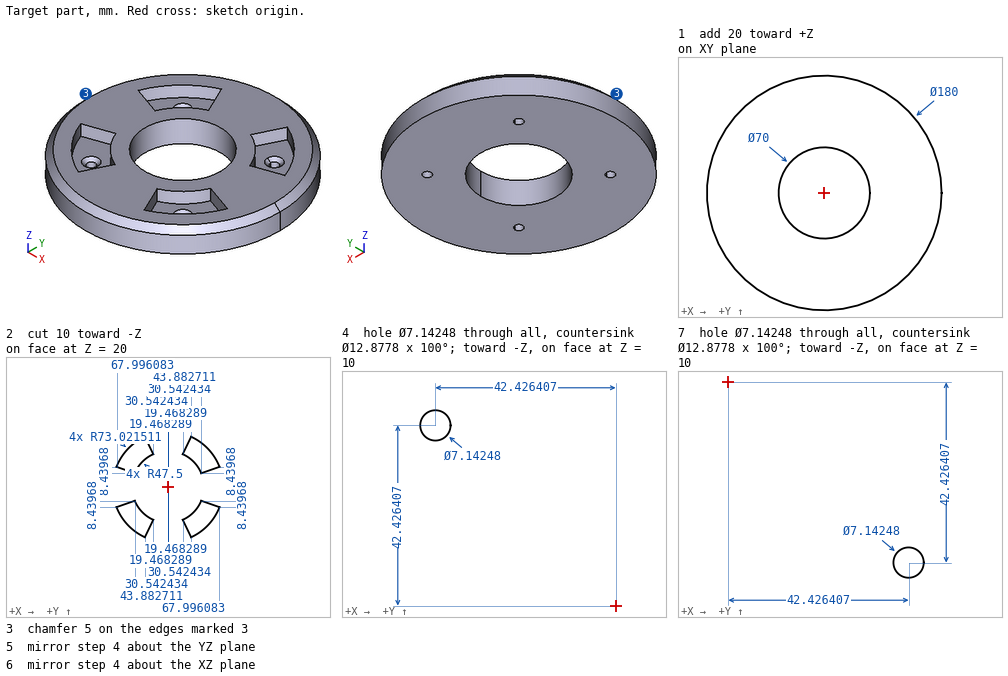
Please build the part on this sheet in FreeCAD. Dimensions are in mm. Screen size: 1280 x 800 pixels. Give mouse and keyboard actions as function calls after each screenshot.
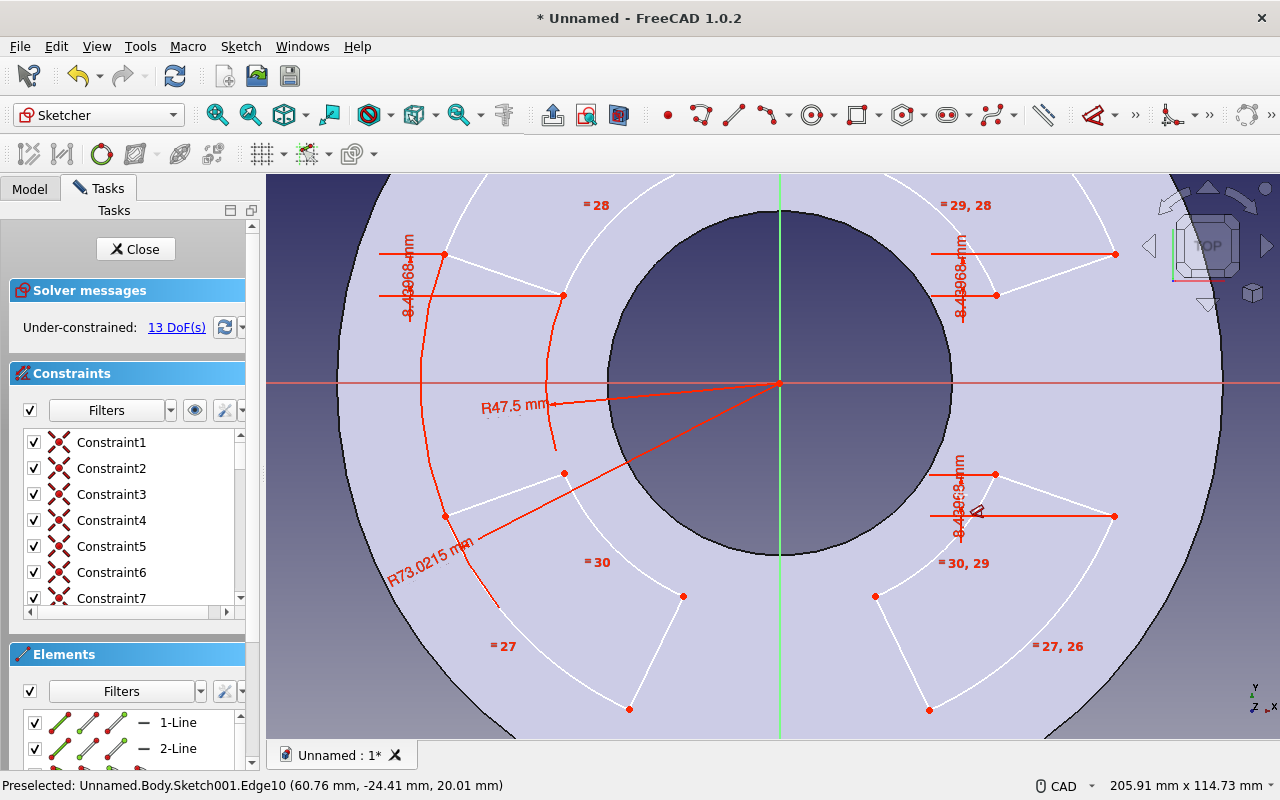
click(529, 487)
click(412, 495)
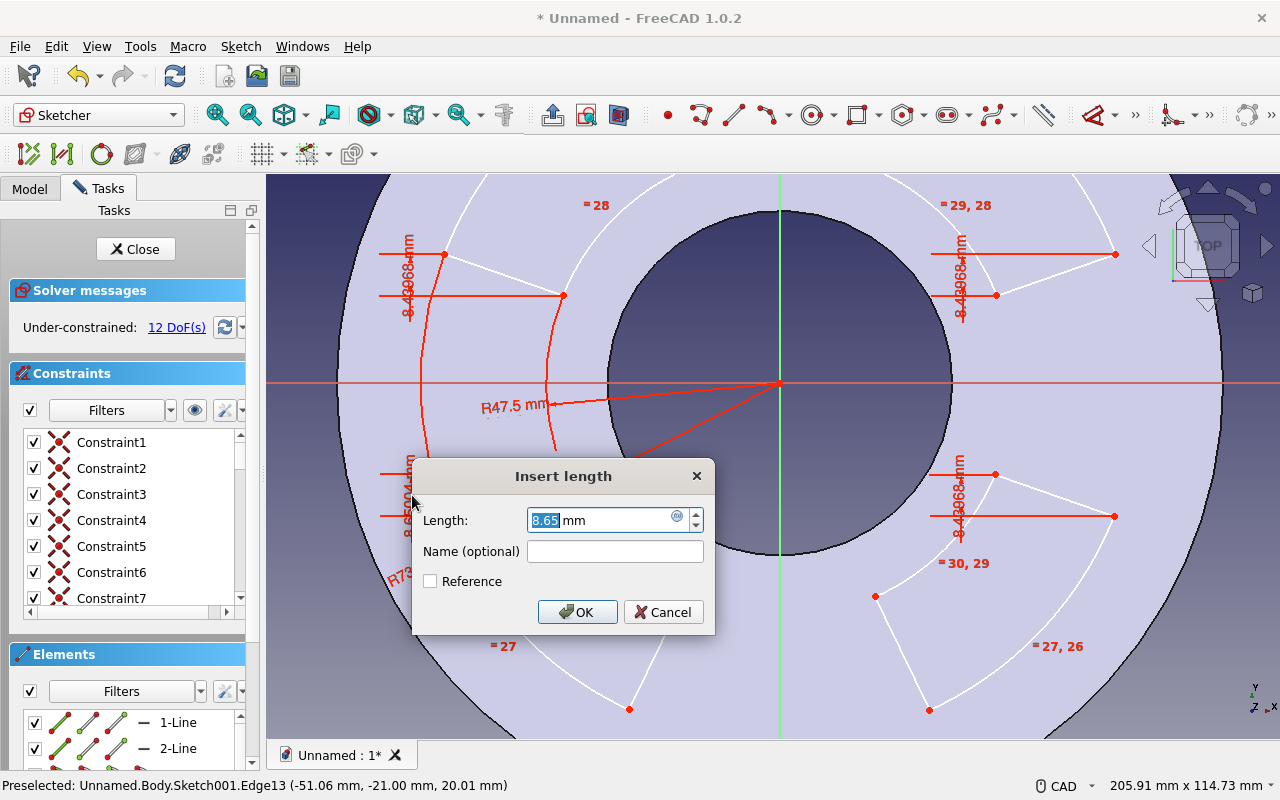
text(8.43968)
key(Return)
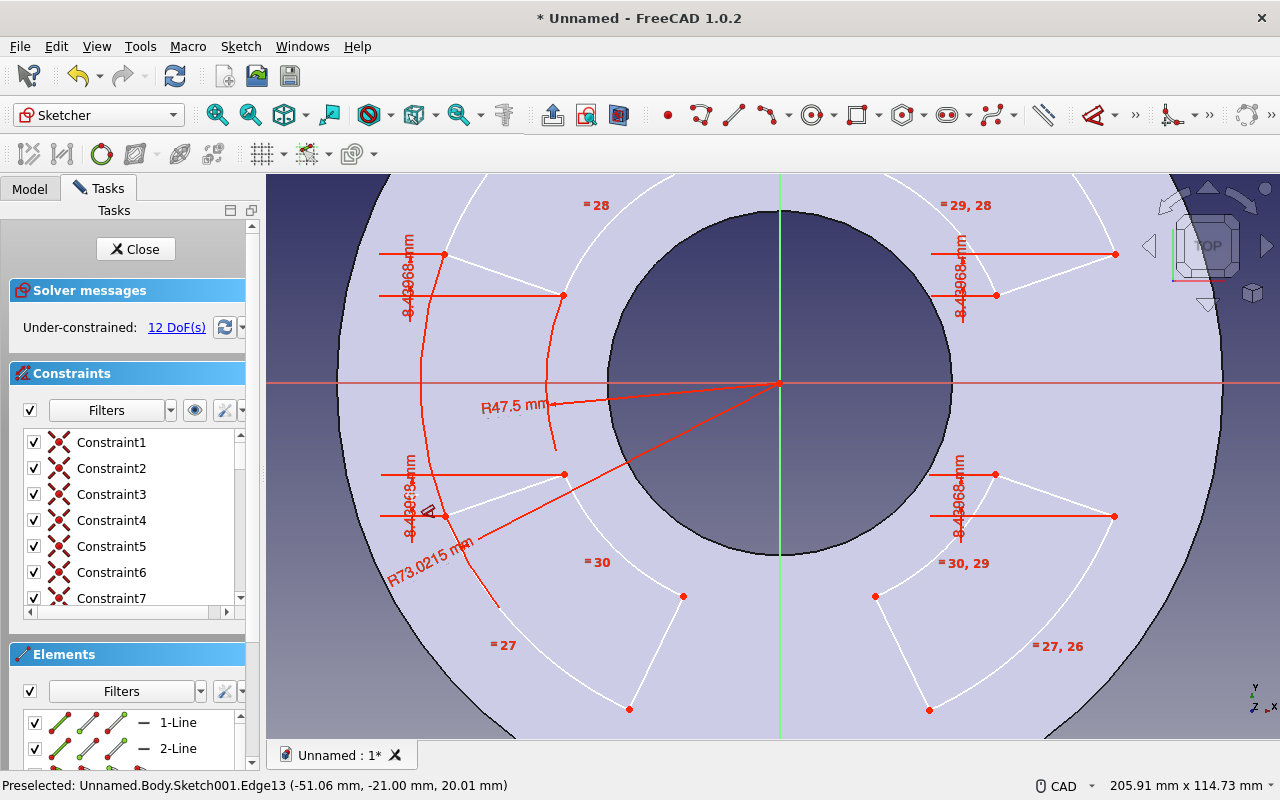
scroll(613, 546, down, 3)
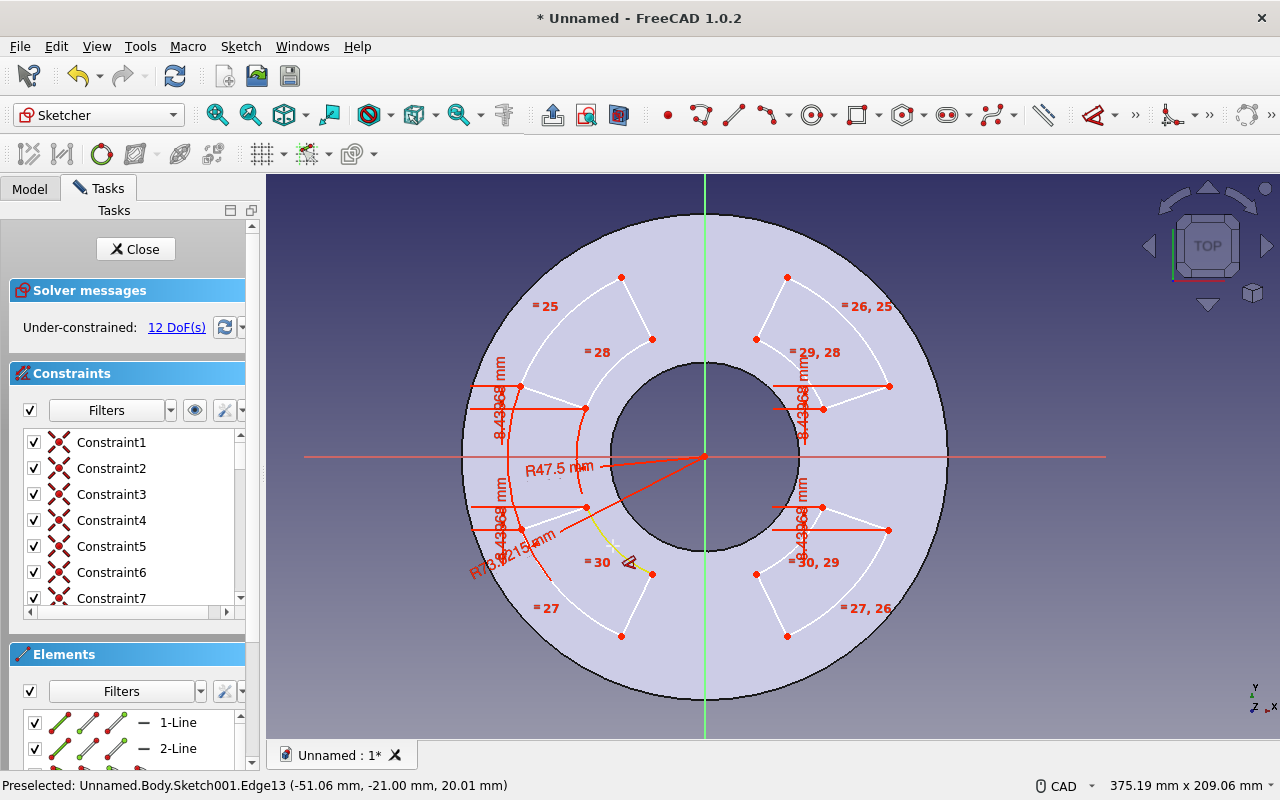
click(652, 340)
click(679, 306)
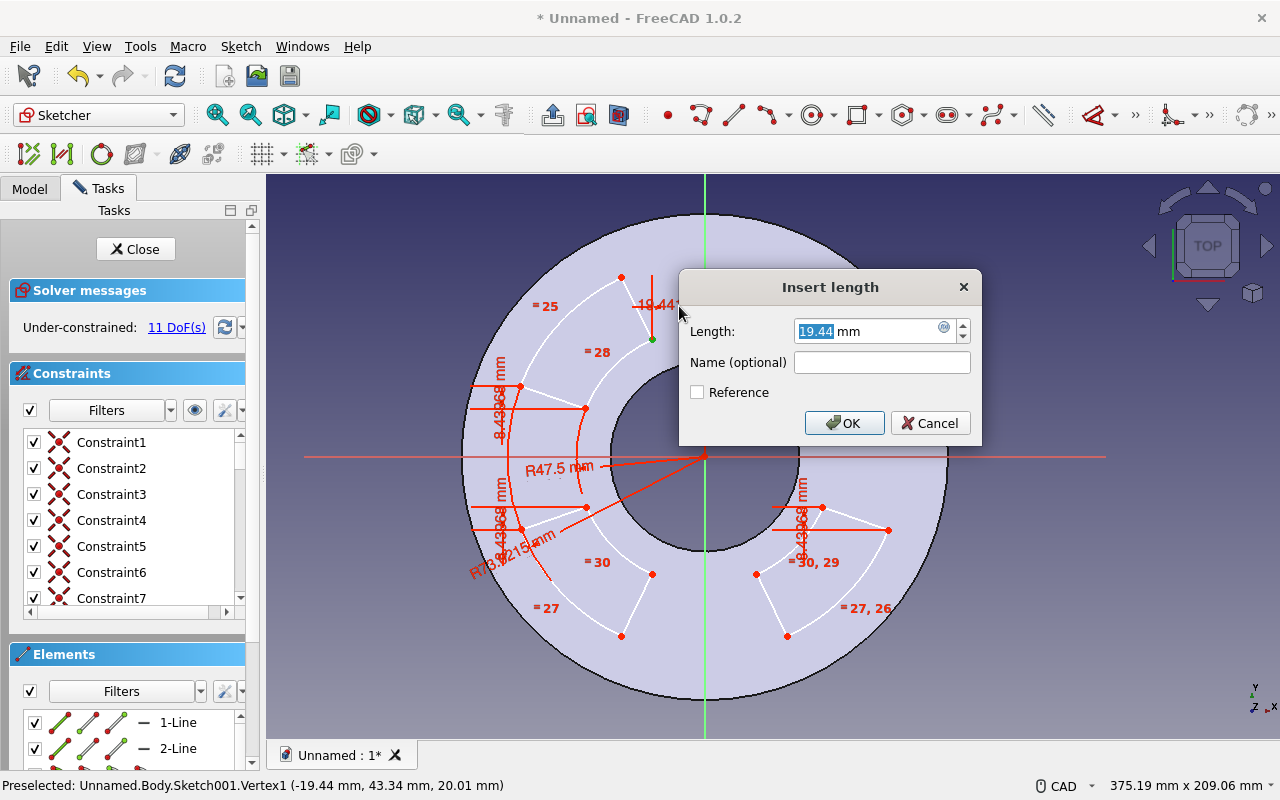
text(19.468289)
key(Return)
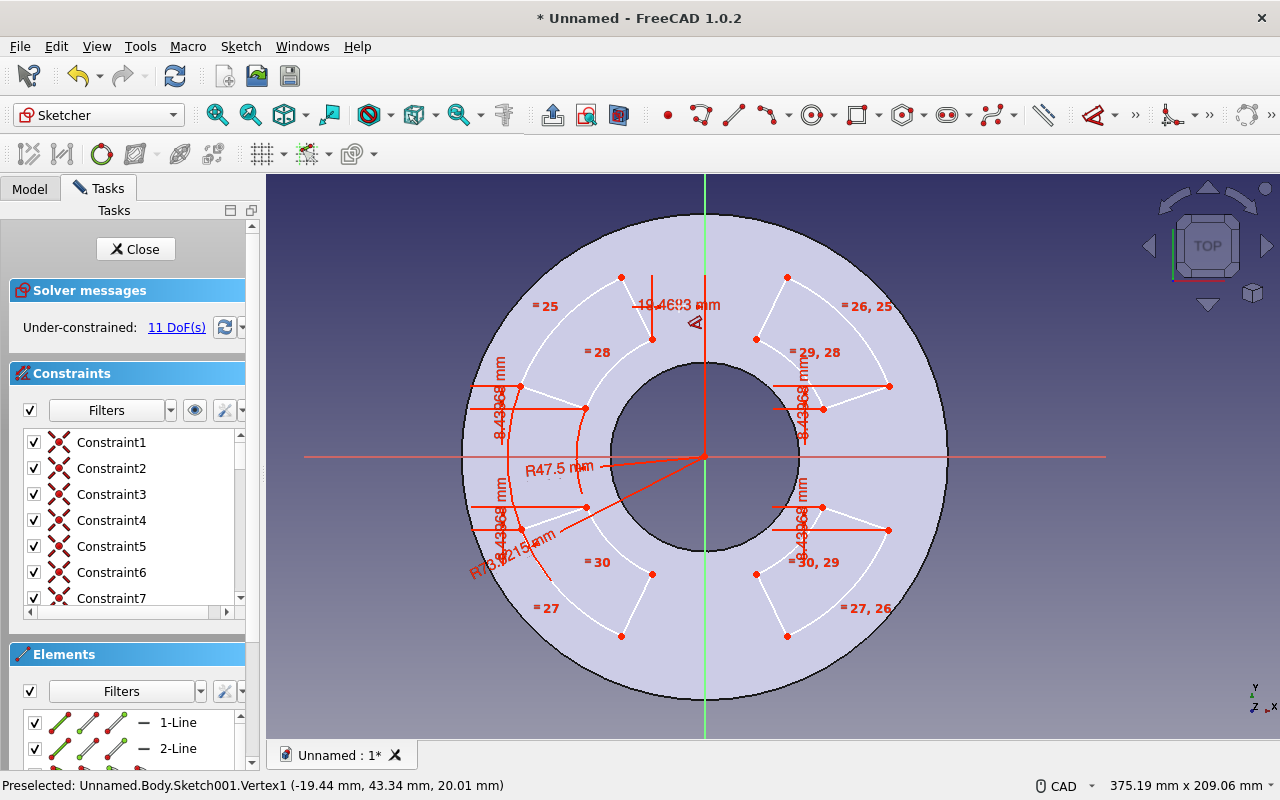
click(622, 278)
click(663, 244)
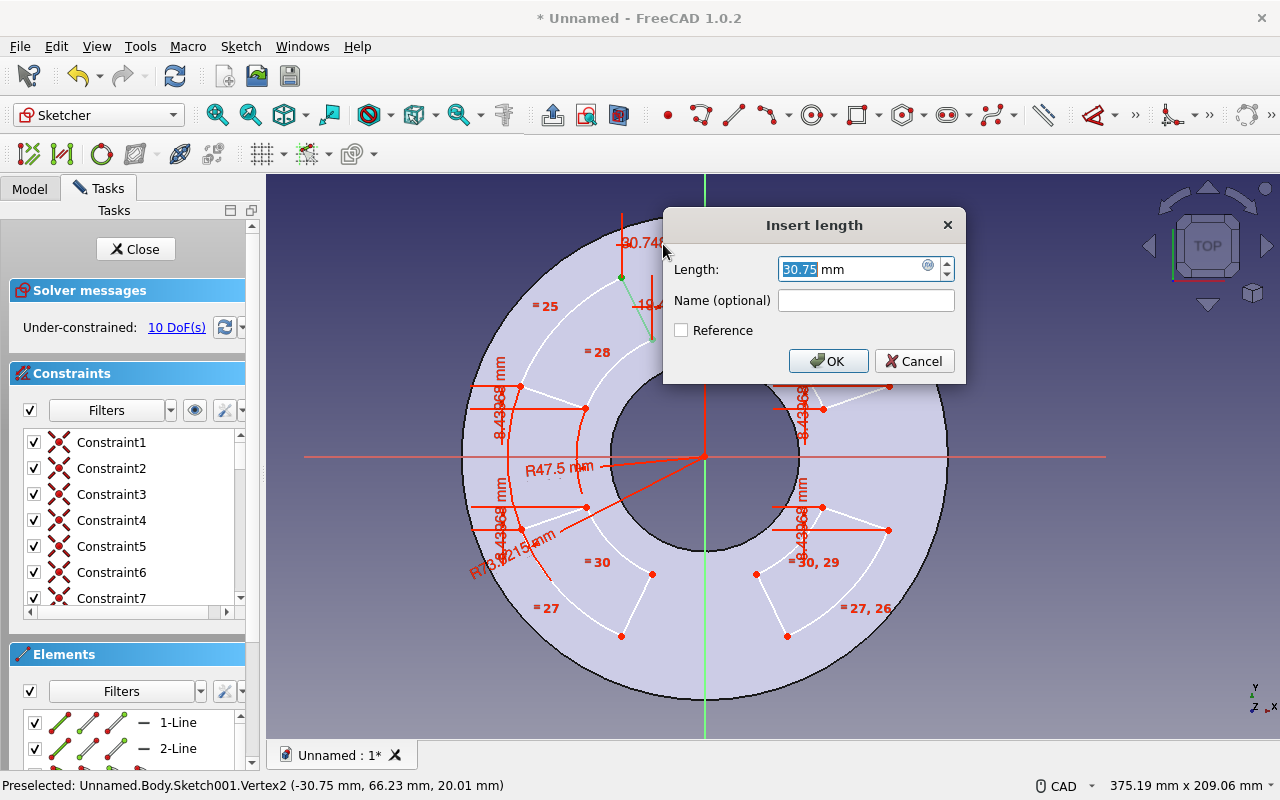
text(30.542434)
key(Return)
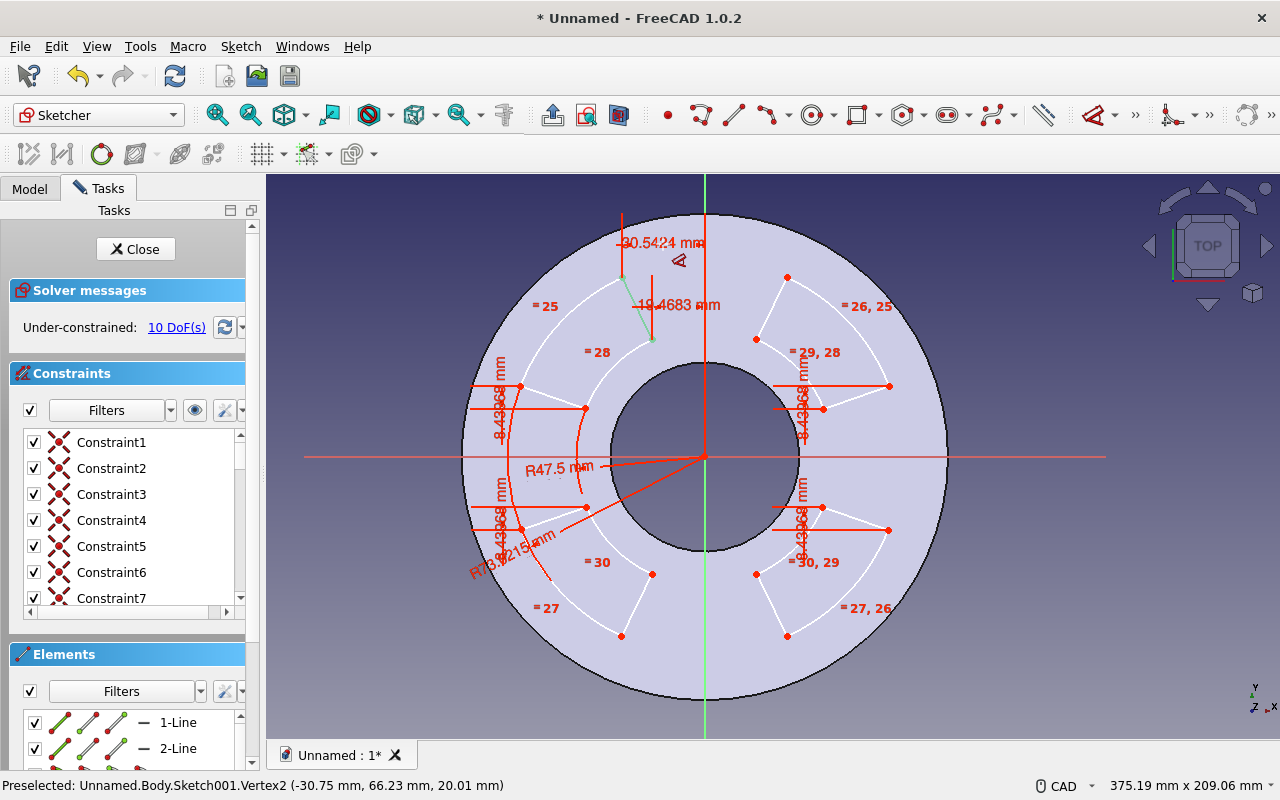
click(521, 386)
click(570, 352)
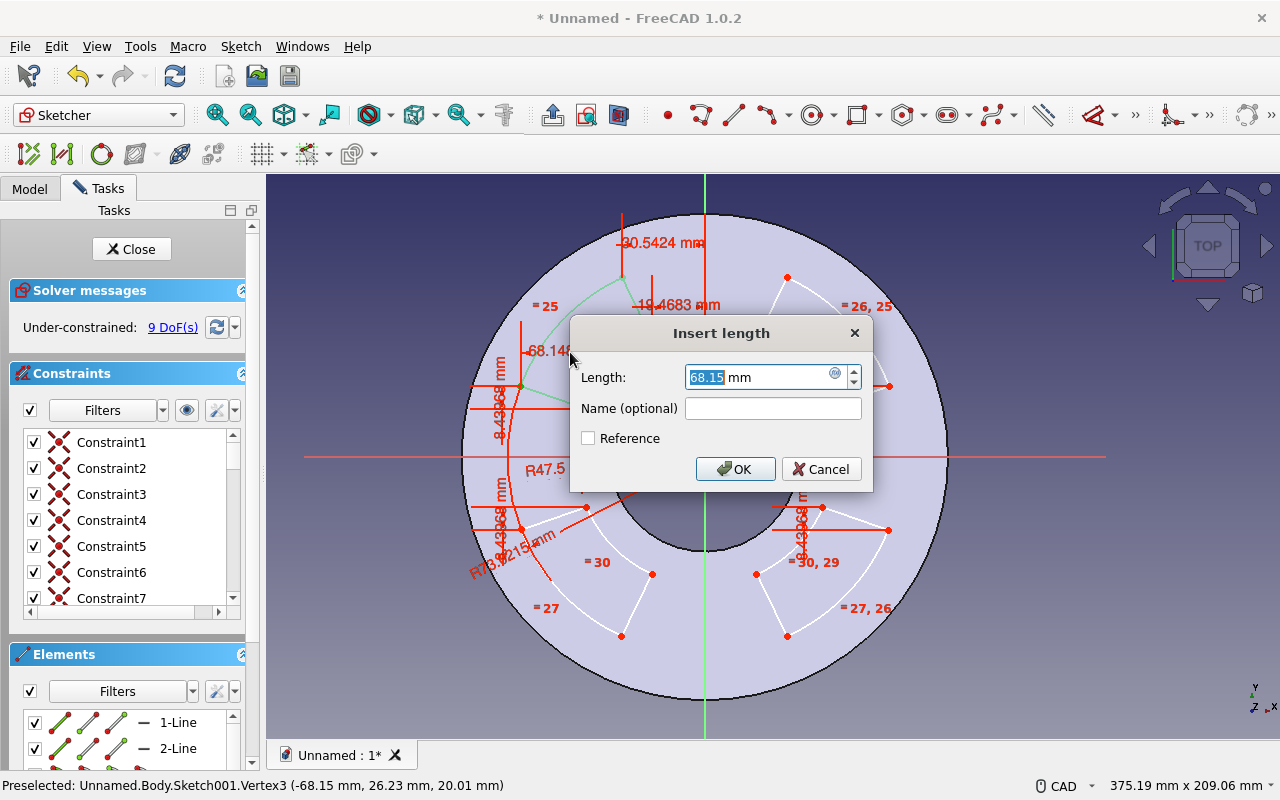
text(67.996083)
key(Return)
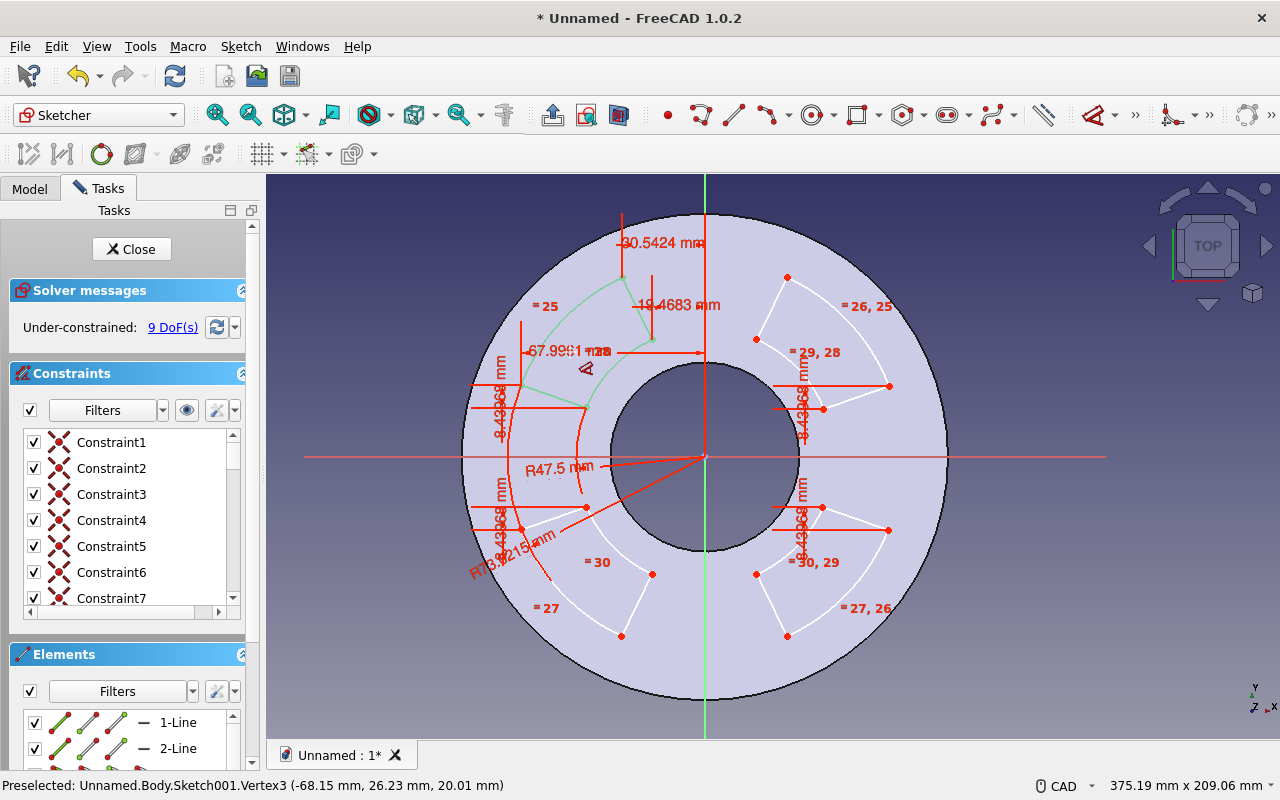
click(824, 409)
click(764, 375)